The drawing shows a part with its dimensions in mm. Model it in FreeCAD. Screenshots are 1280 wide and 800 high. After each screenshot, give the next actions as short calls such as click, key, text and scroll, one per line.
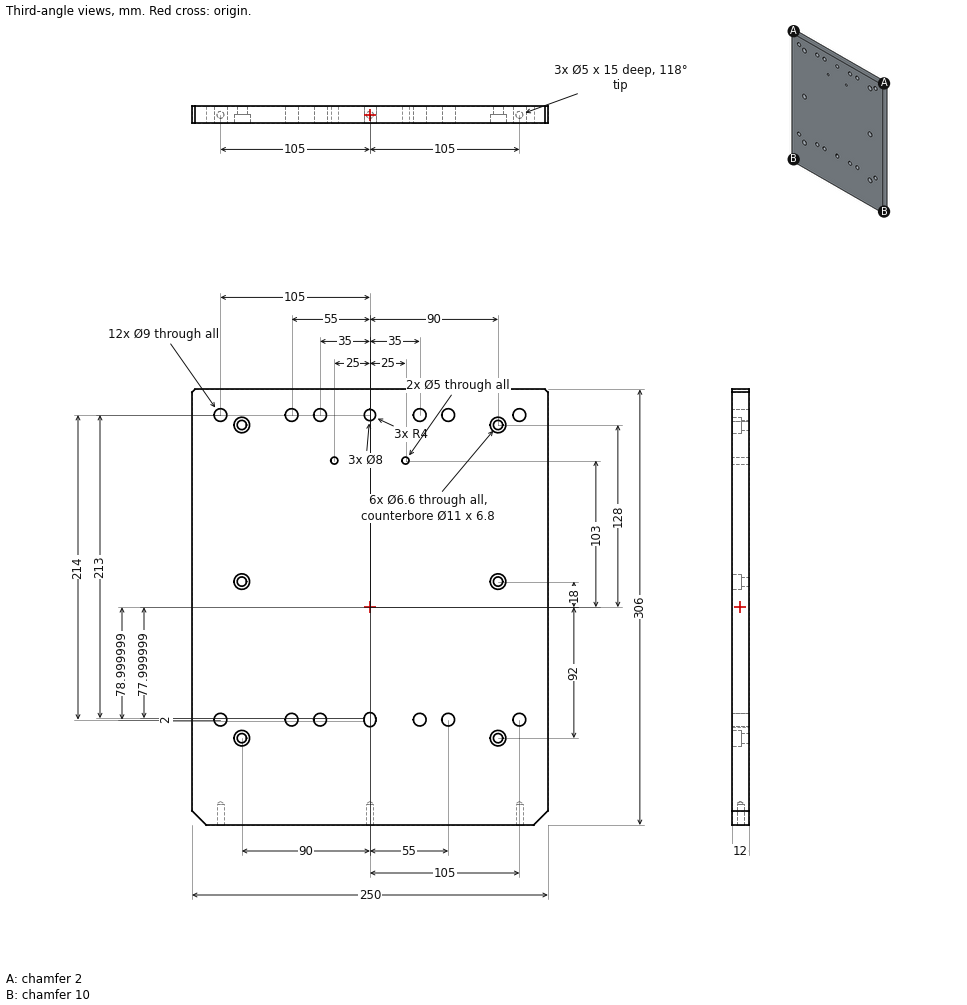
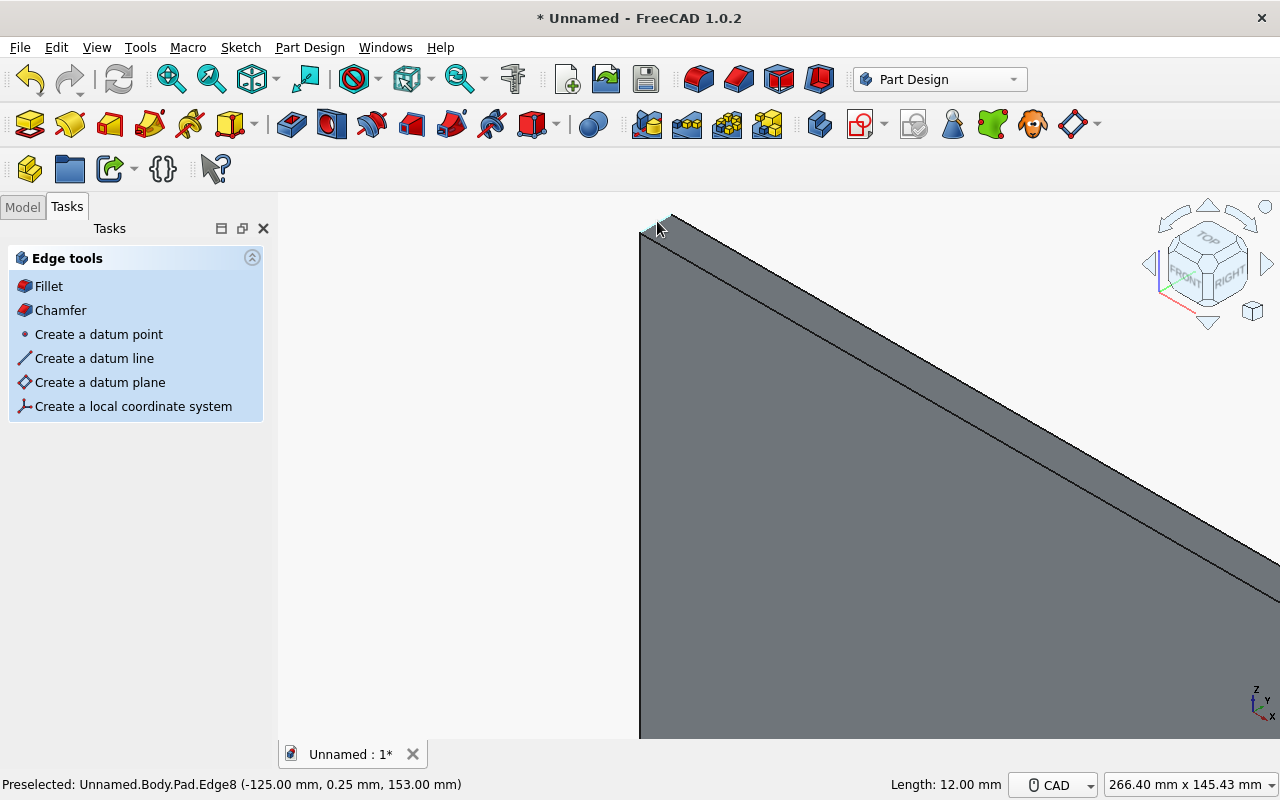
click(172, 80)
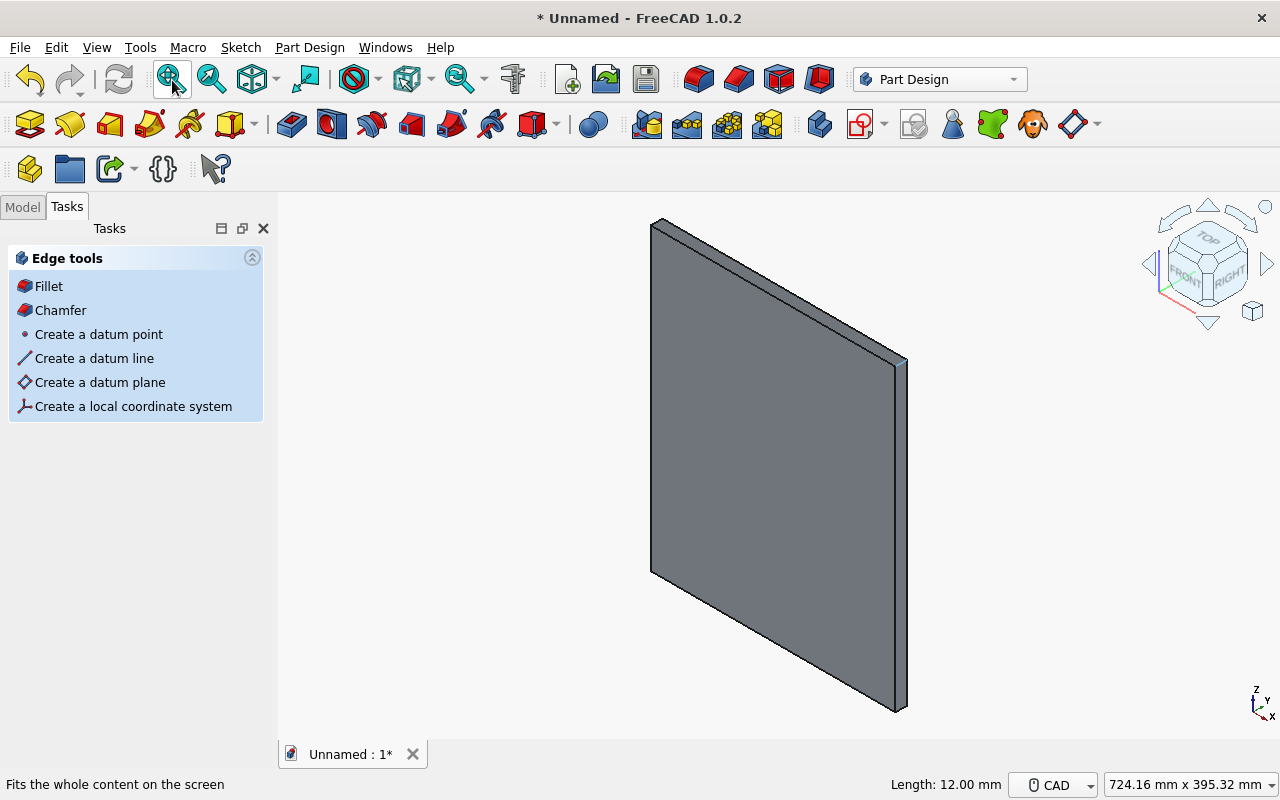
key(2)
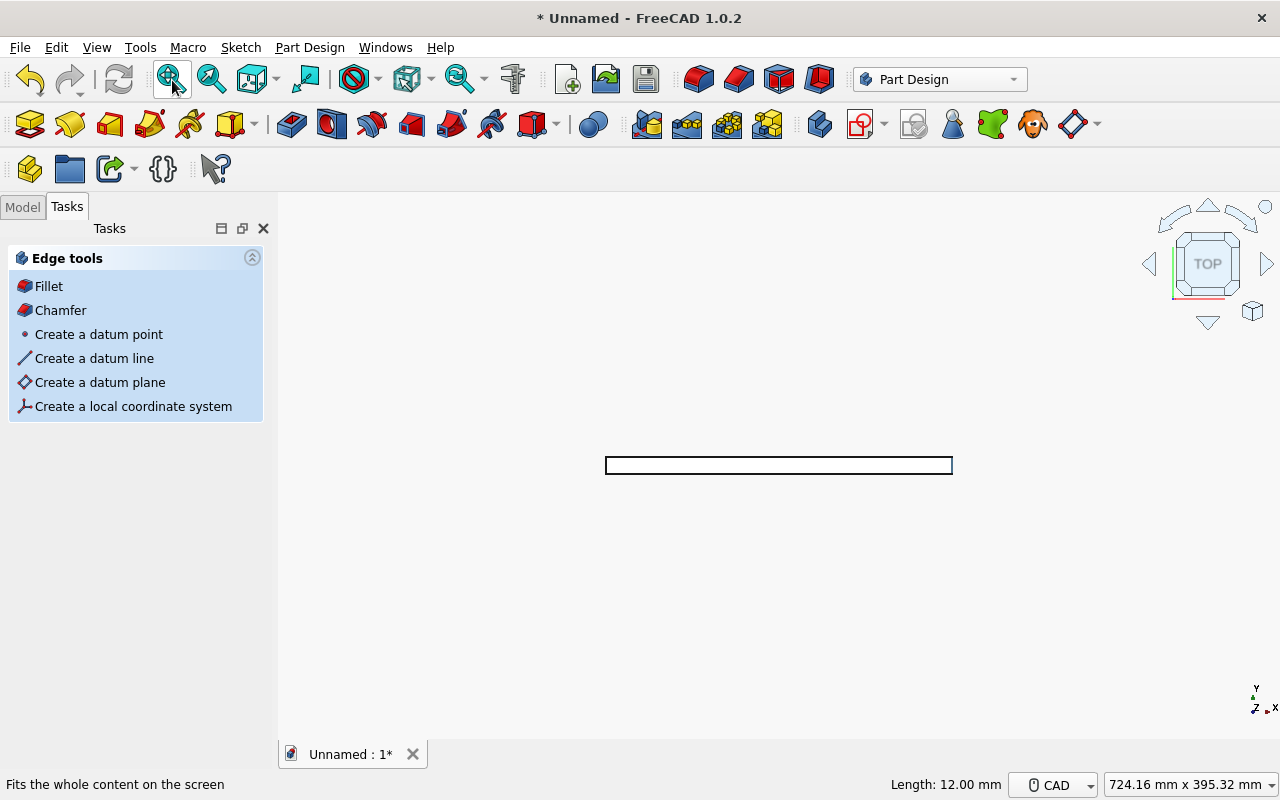
key(v)
key(f)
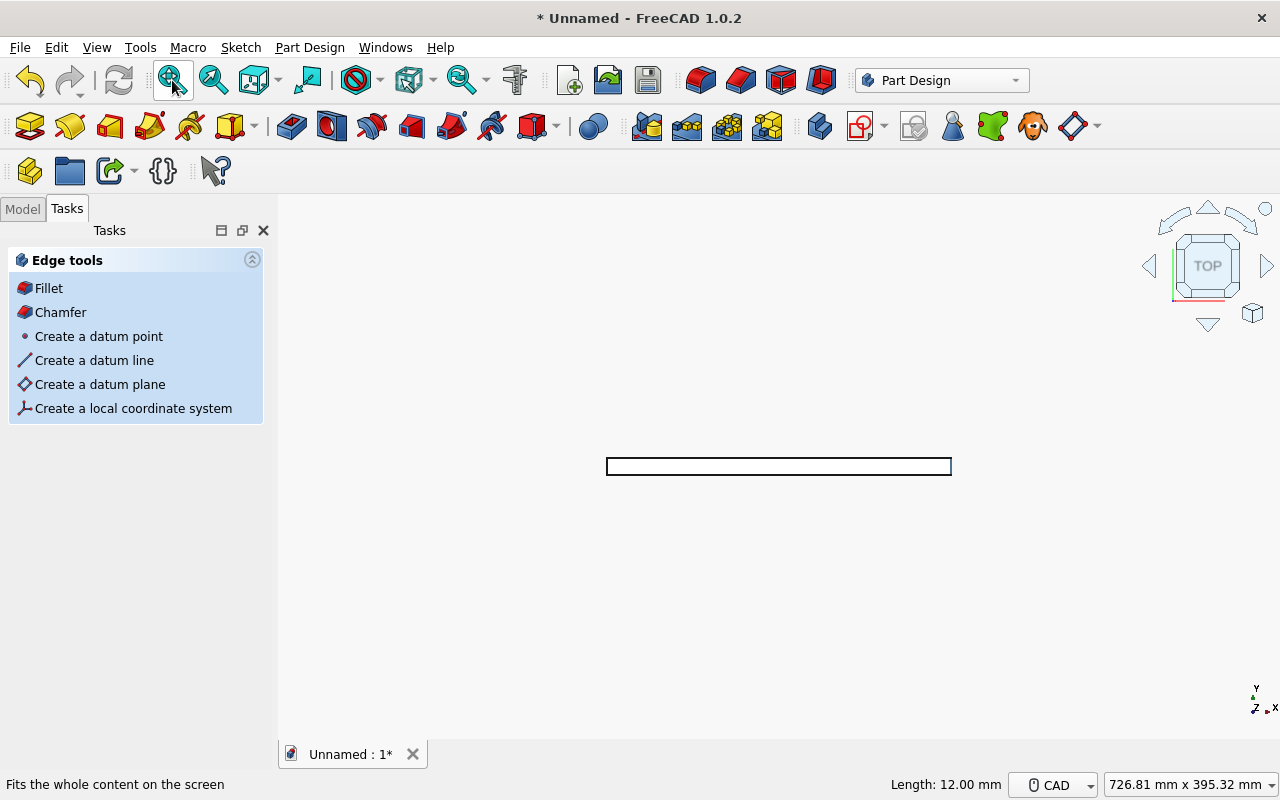
click(607, 465, ctrl)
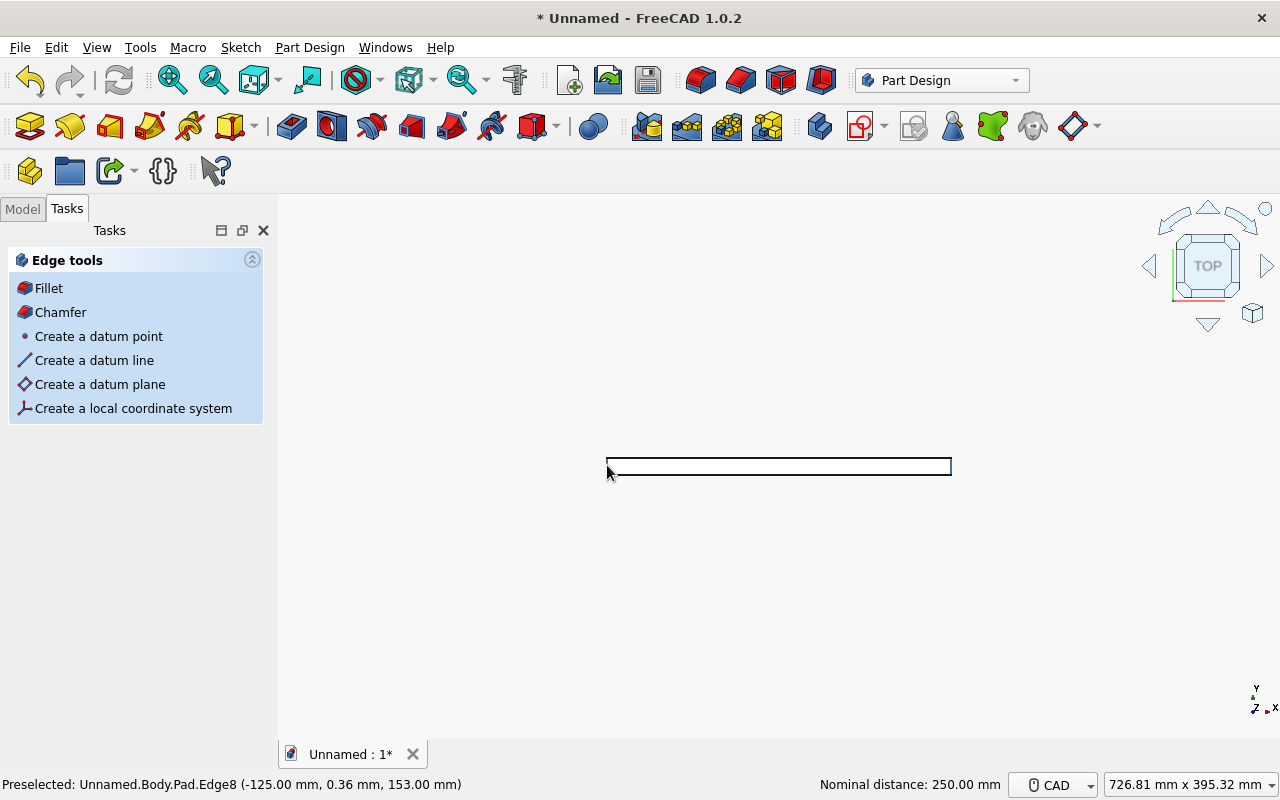
click(742, 80)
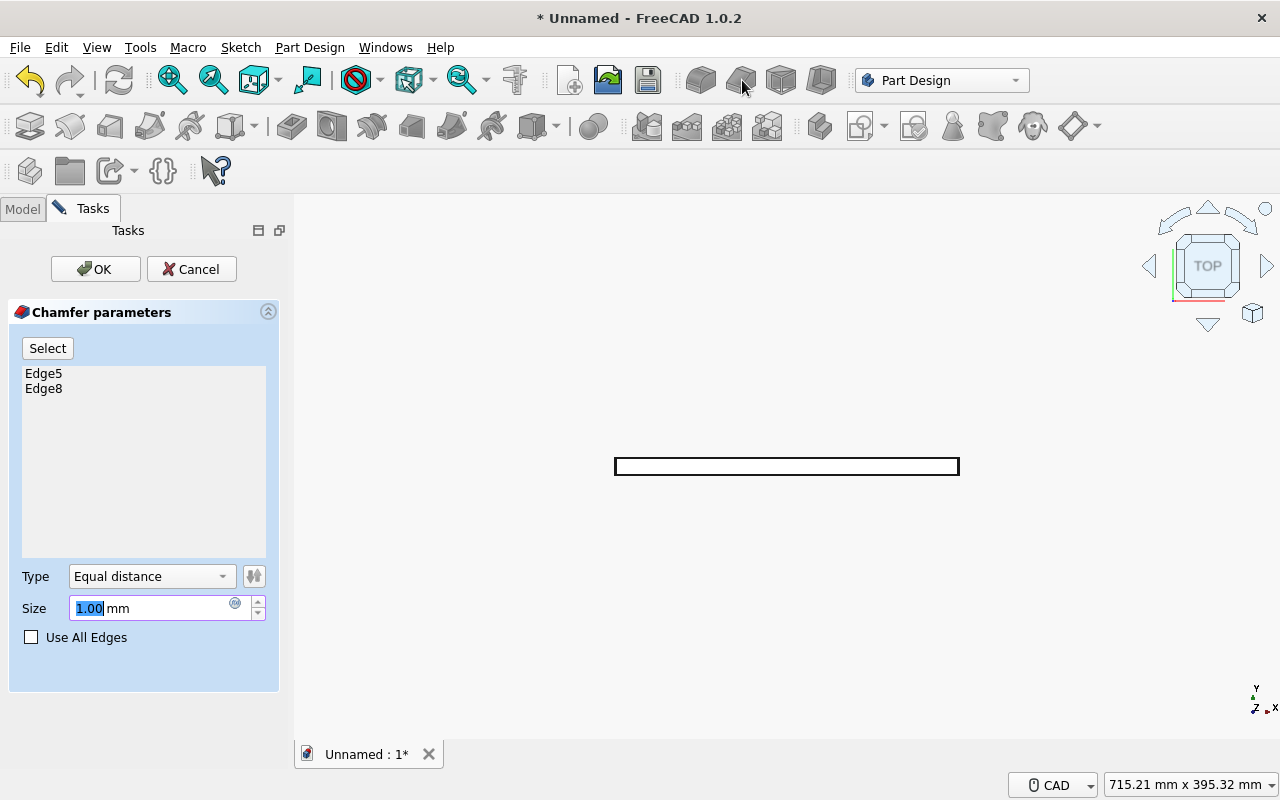
text(2)
key(Tab)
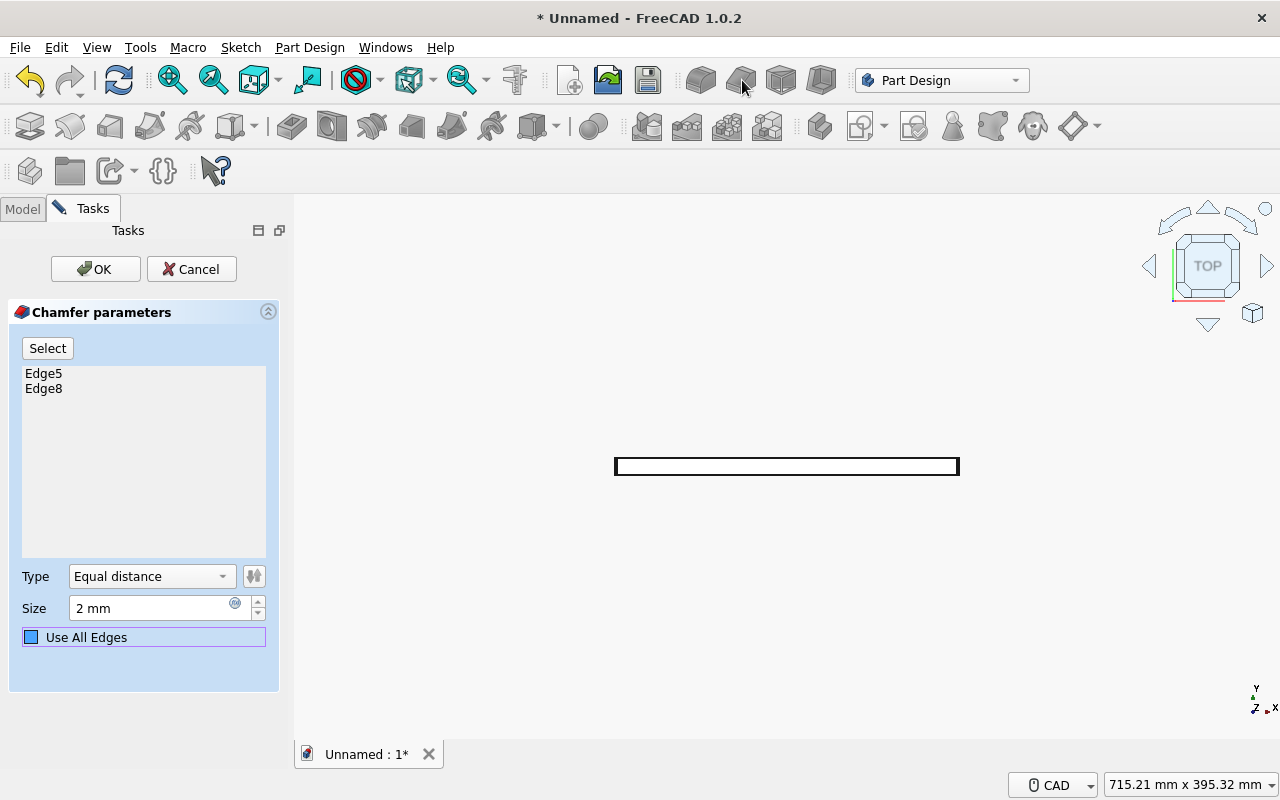
click(96, 269)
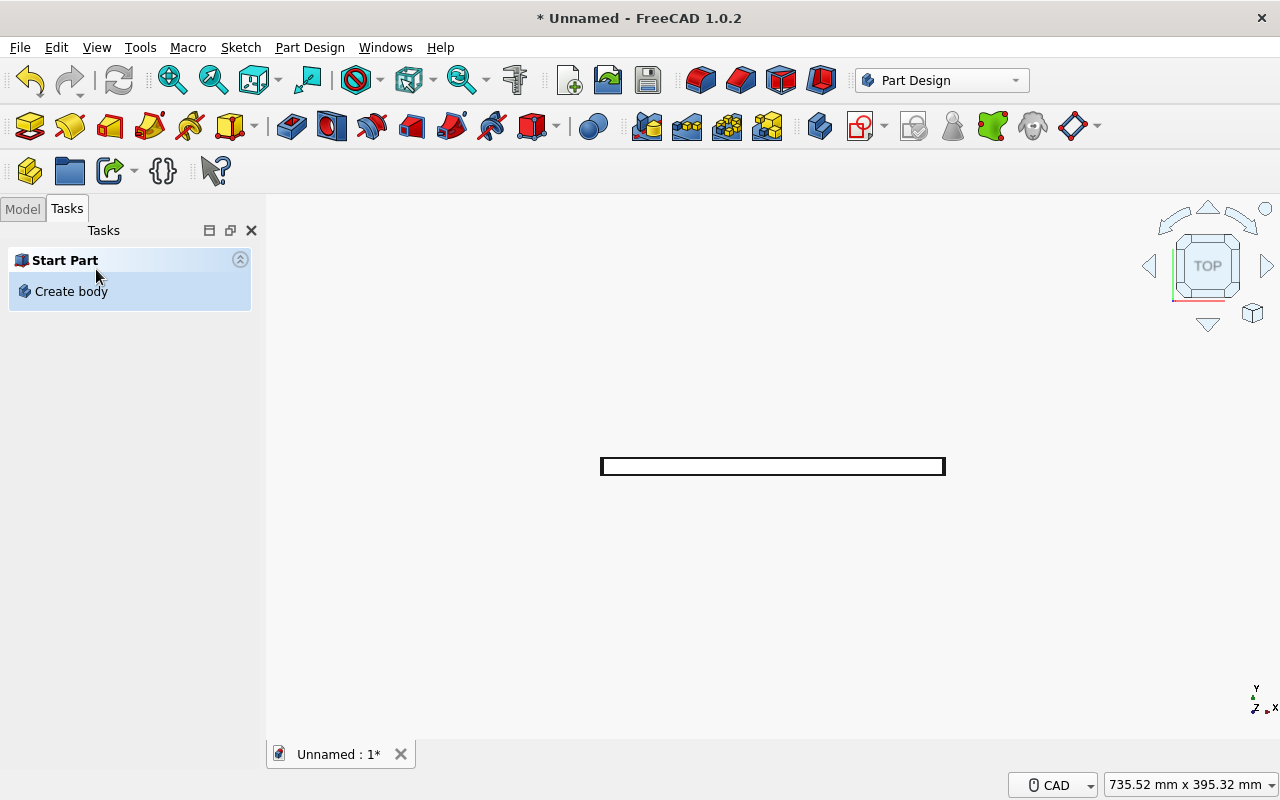
click(174, 80)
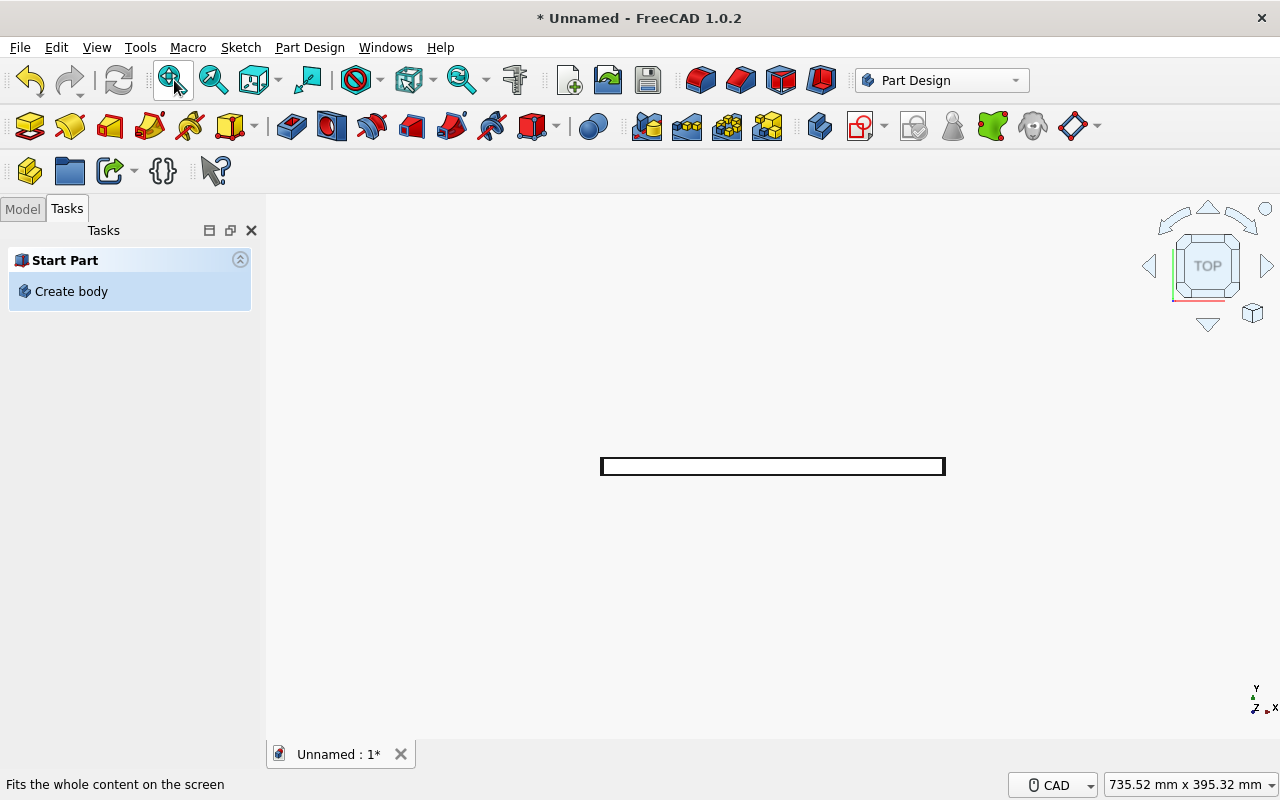
key(5)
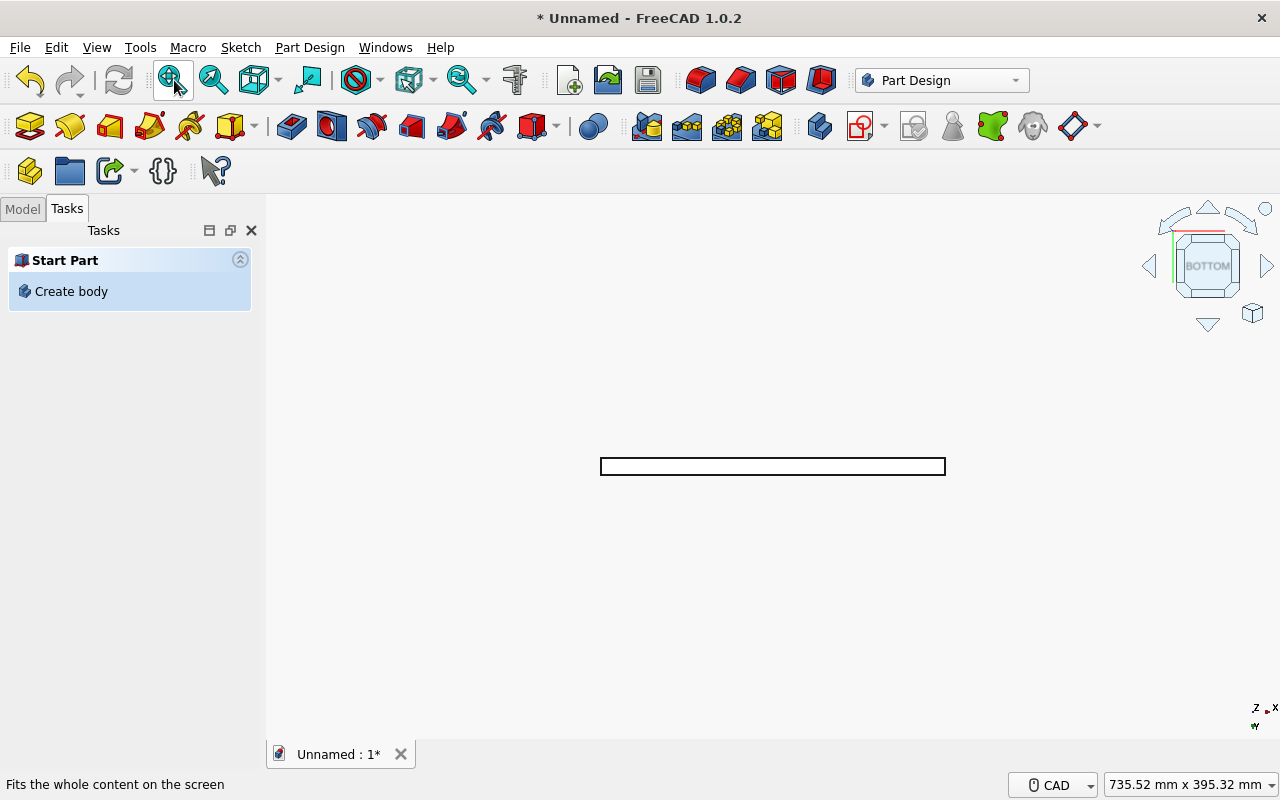
click(174, 80)